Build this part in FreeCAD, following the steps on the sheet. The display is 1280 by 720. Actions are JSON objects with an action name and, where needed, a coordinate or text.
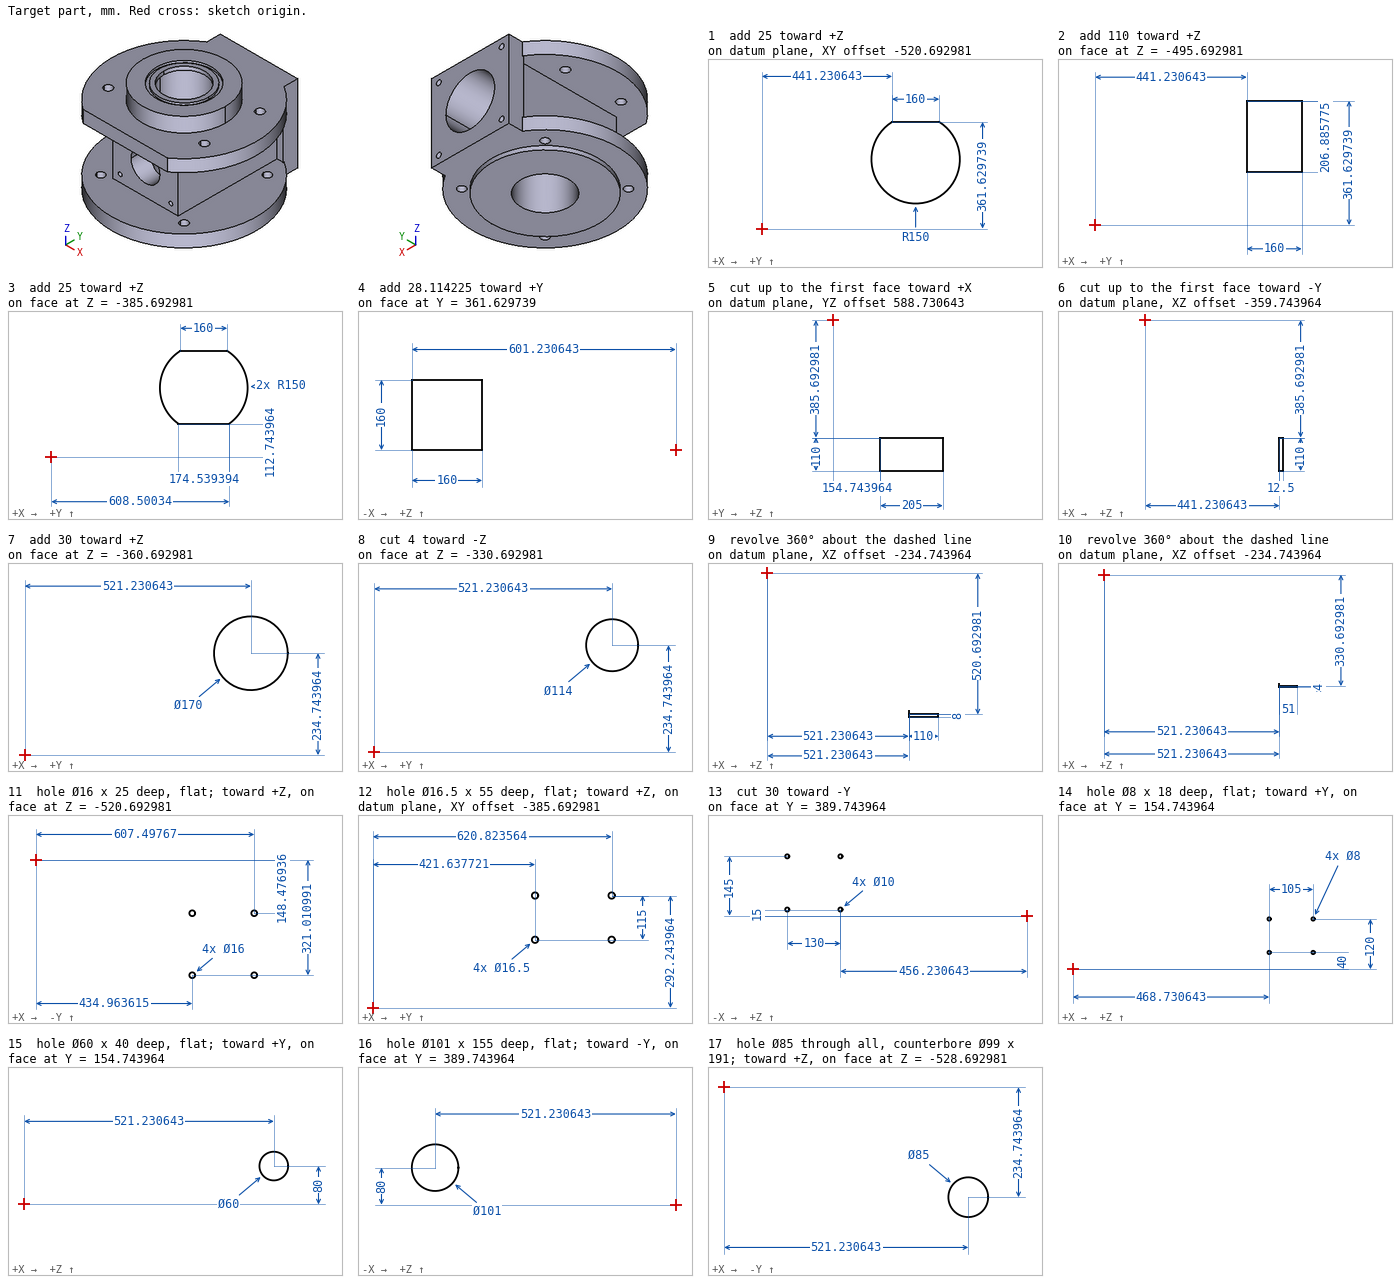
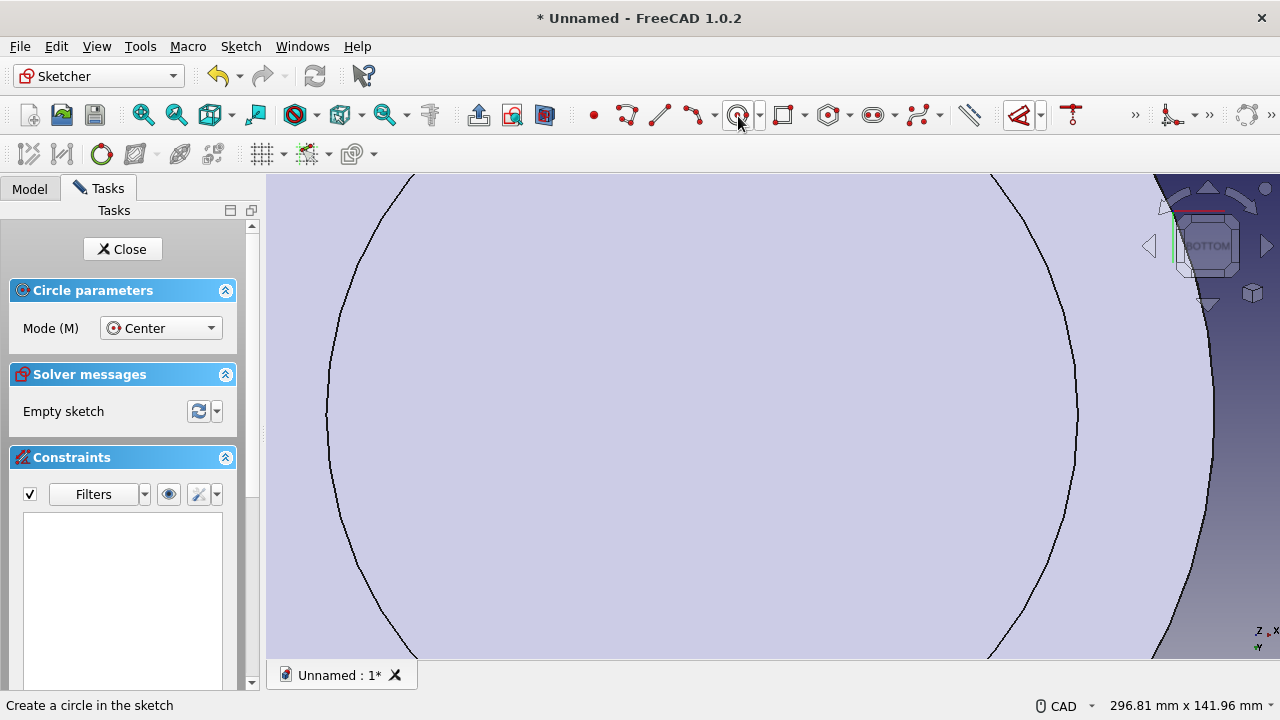
{"action": "left_click", "coordinate": [702, 415]}
{"action": "left_click", "coordinate": [805, 312]}
{"action": "key", "text": "Escape"}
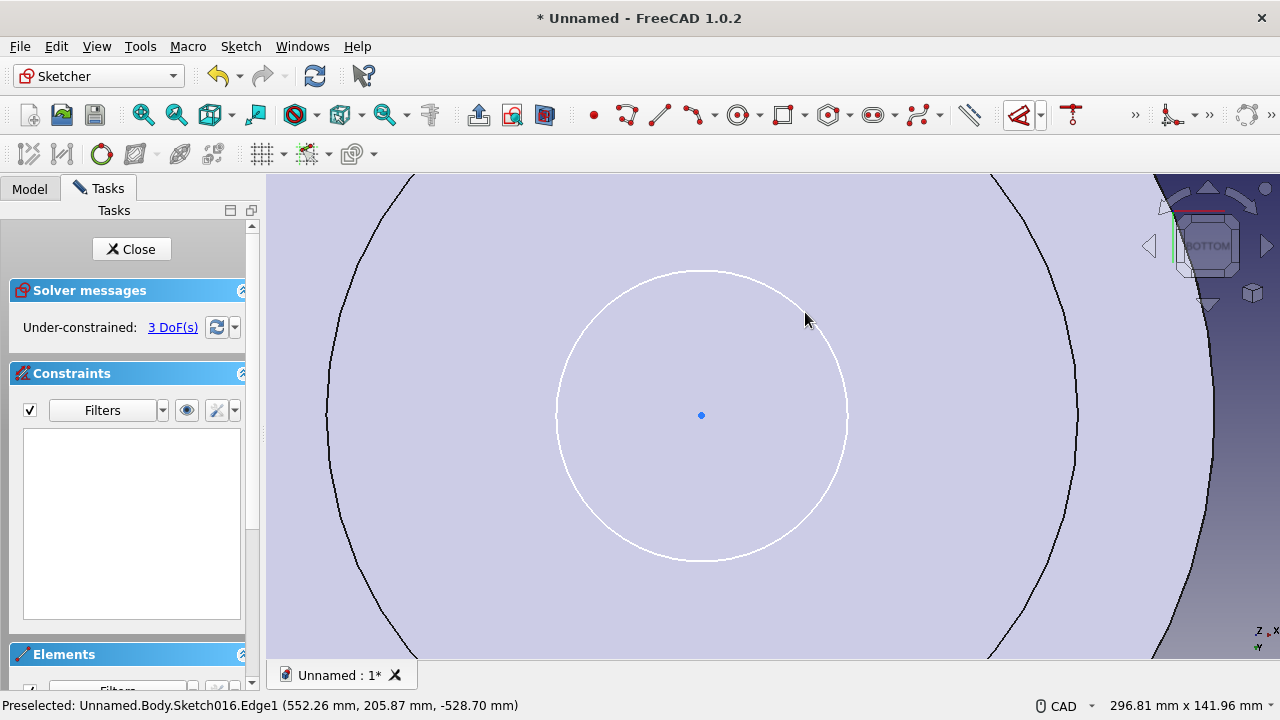
{"action": "left_click", "coordinate": [805, 313]}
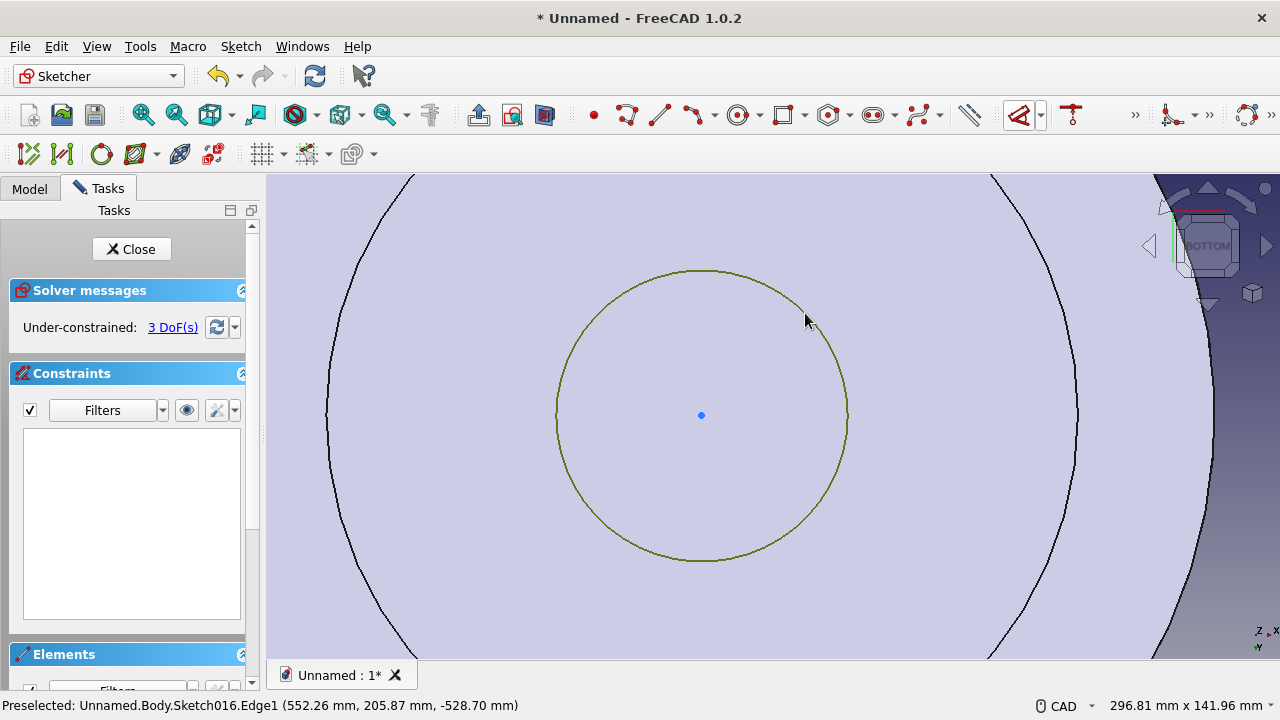
{"action": "key", "text": "k o"}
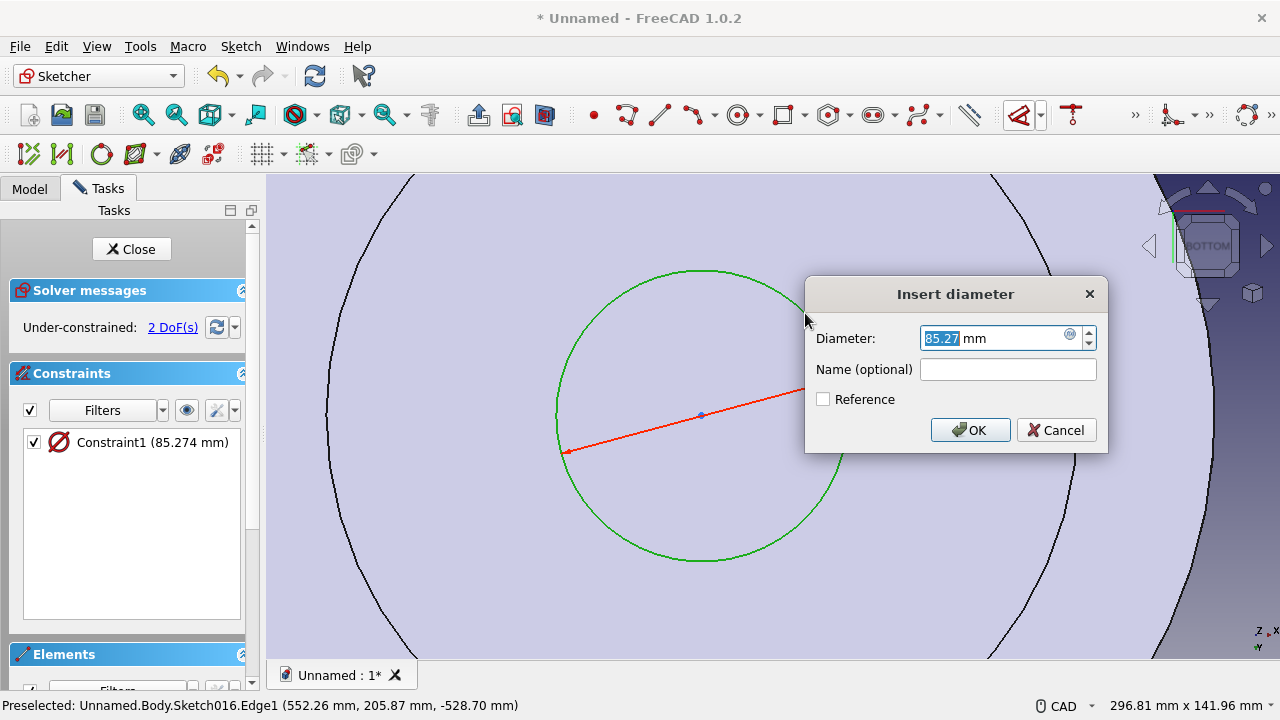
{"action": "type", "text": "85"}
{"action": "key", "text": "Return"}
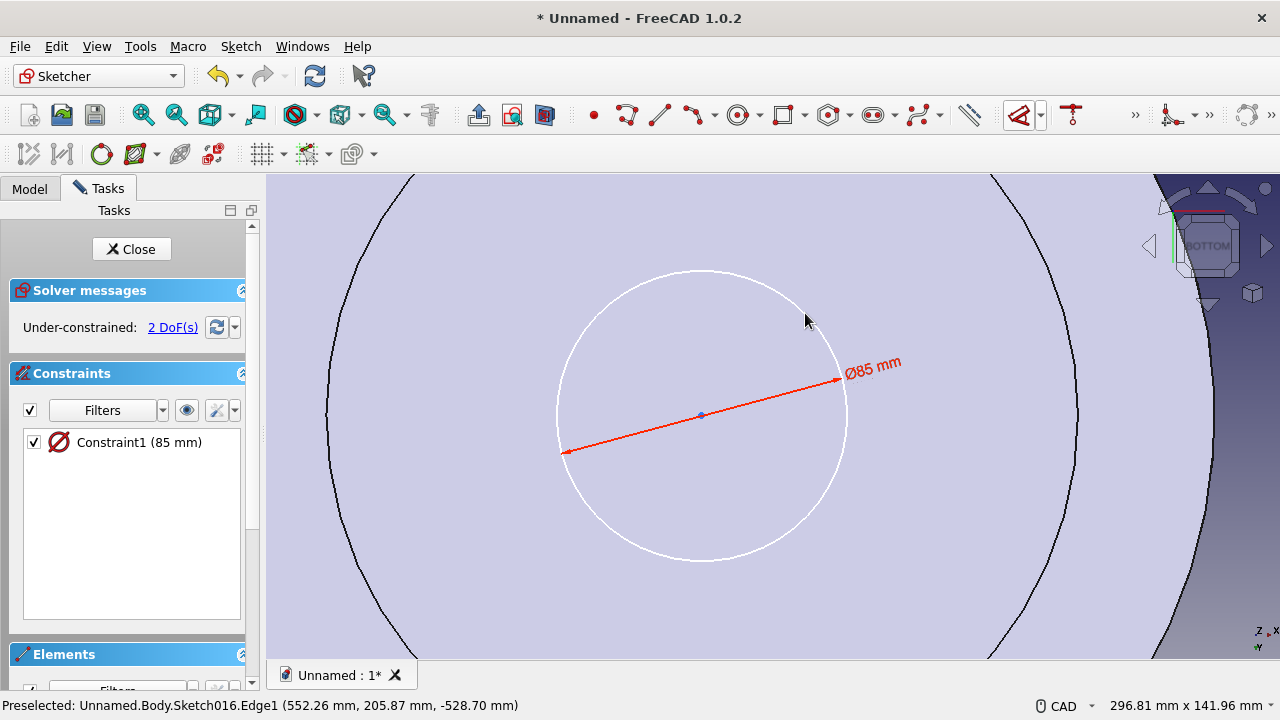
{"action": "left_click", "coordinate": [702, 416]}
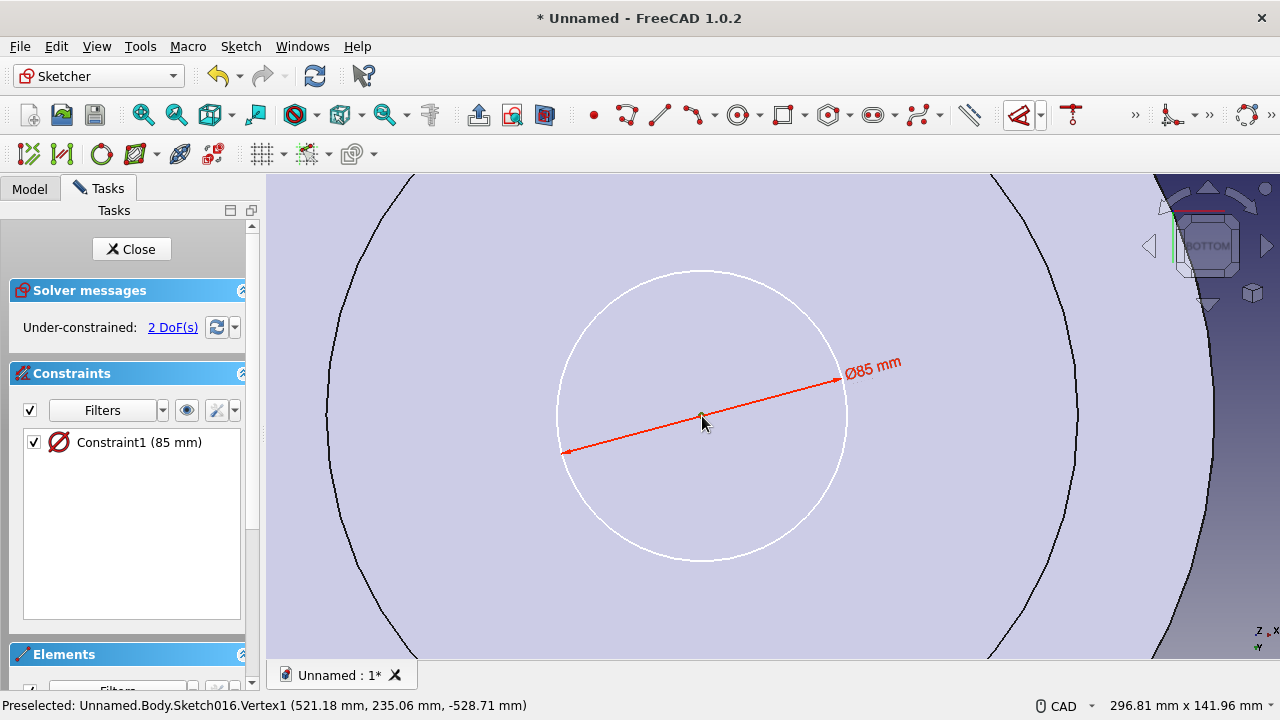
{"action": "key", "text": "l"}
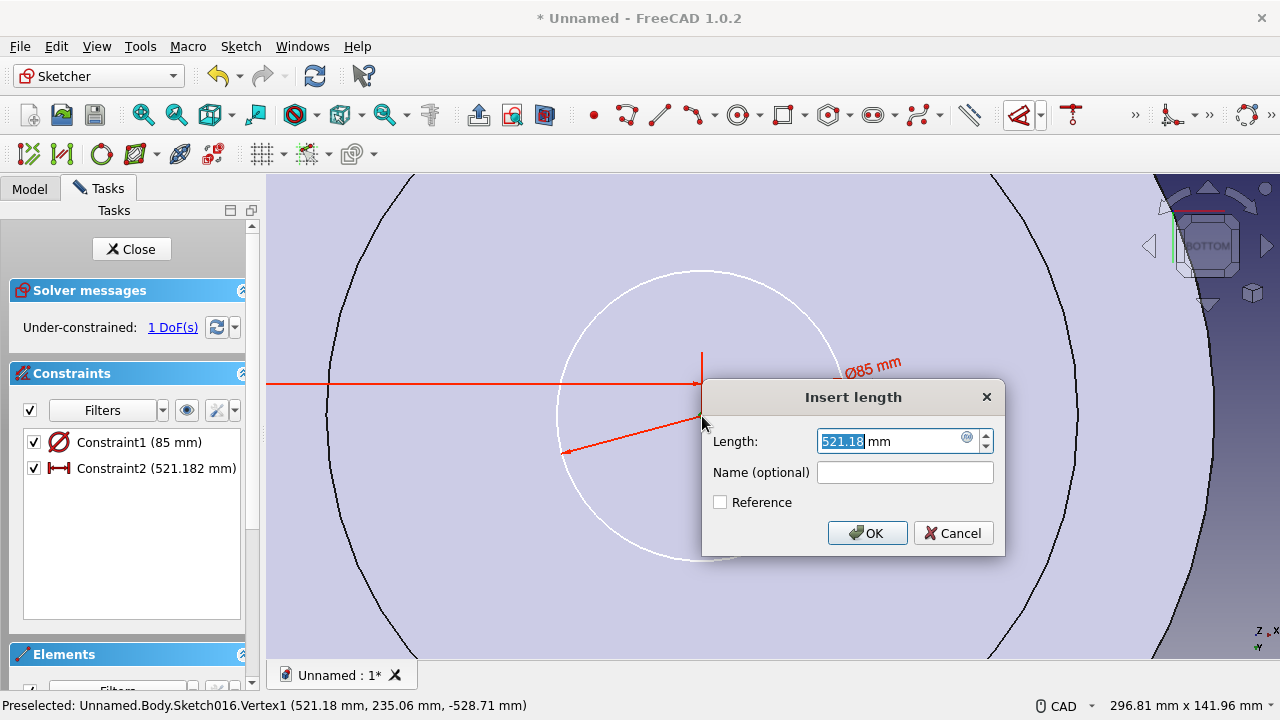
{"action": "type", "text": "521.230643"}
{"action": "key", "text": "Return"}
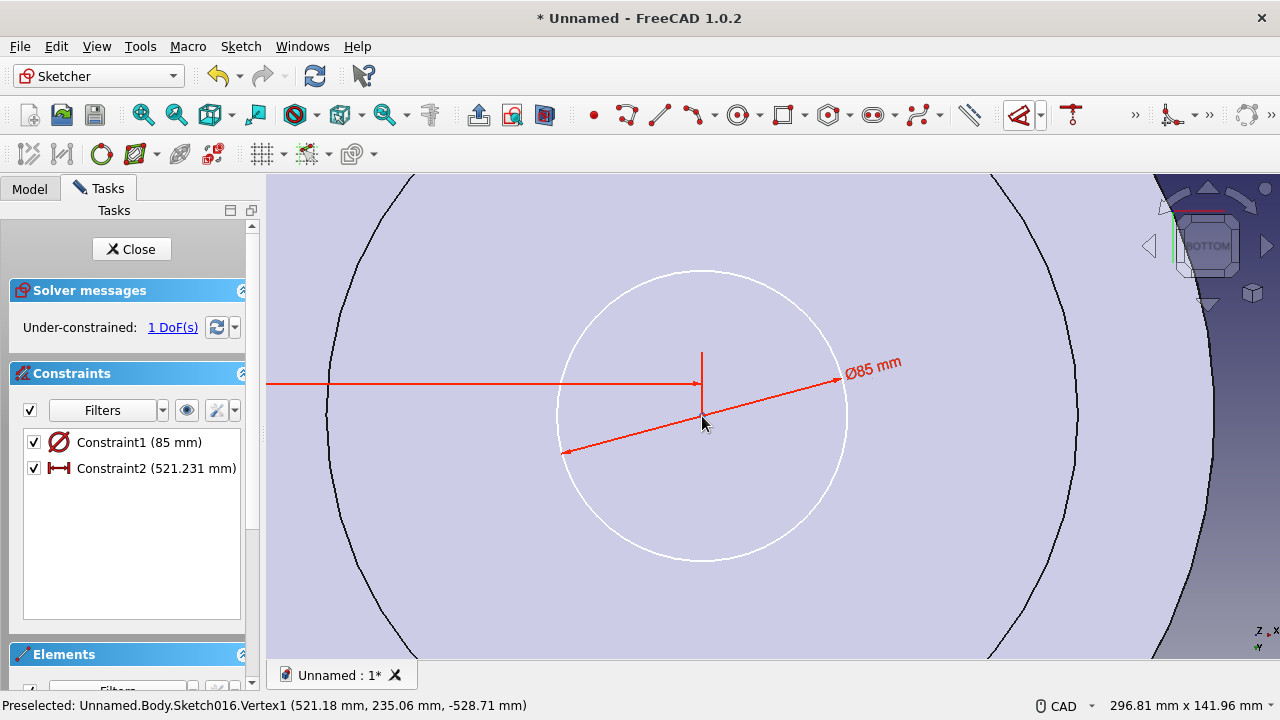
{"action": "left_click", "coordinate": [702, 416]}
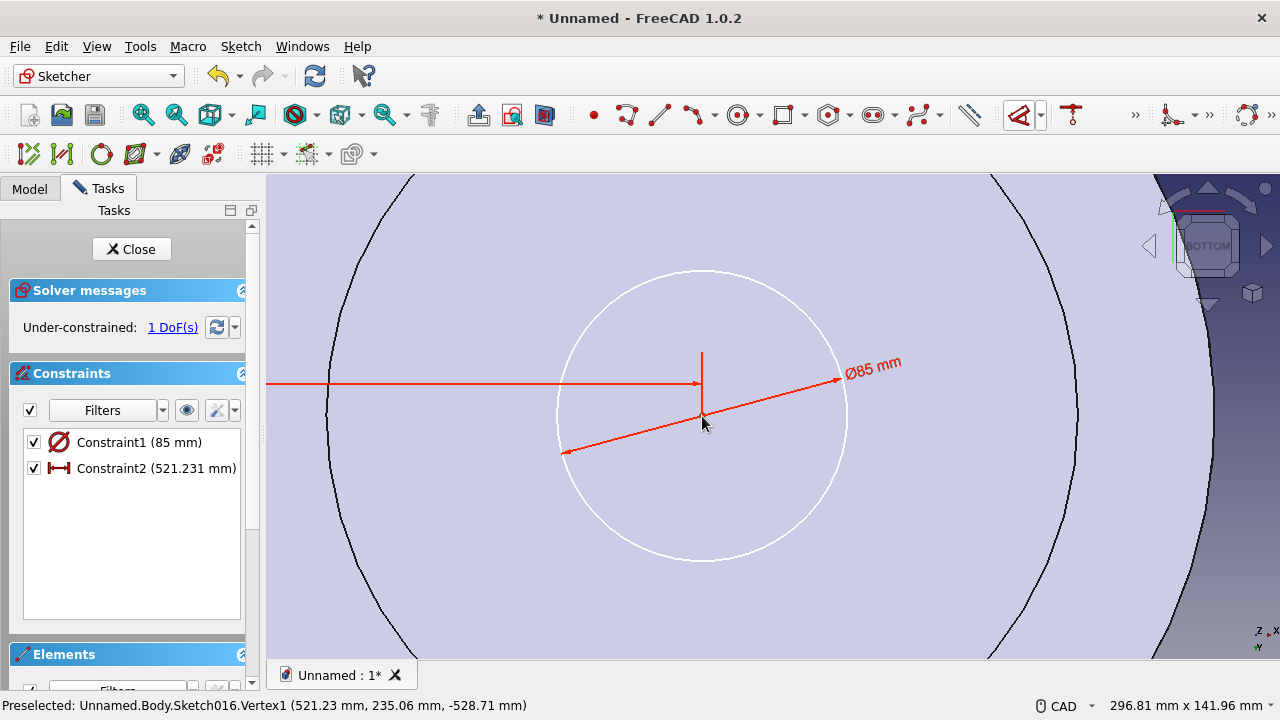
{"action": "left_click", "coordinate": [1040, 116]}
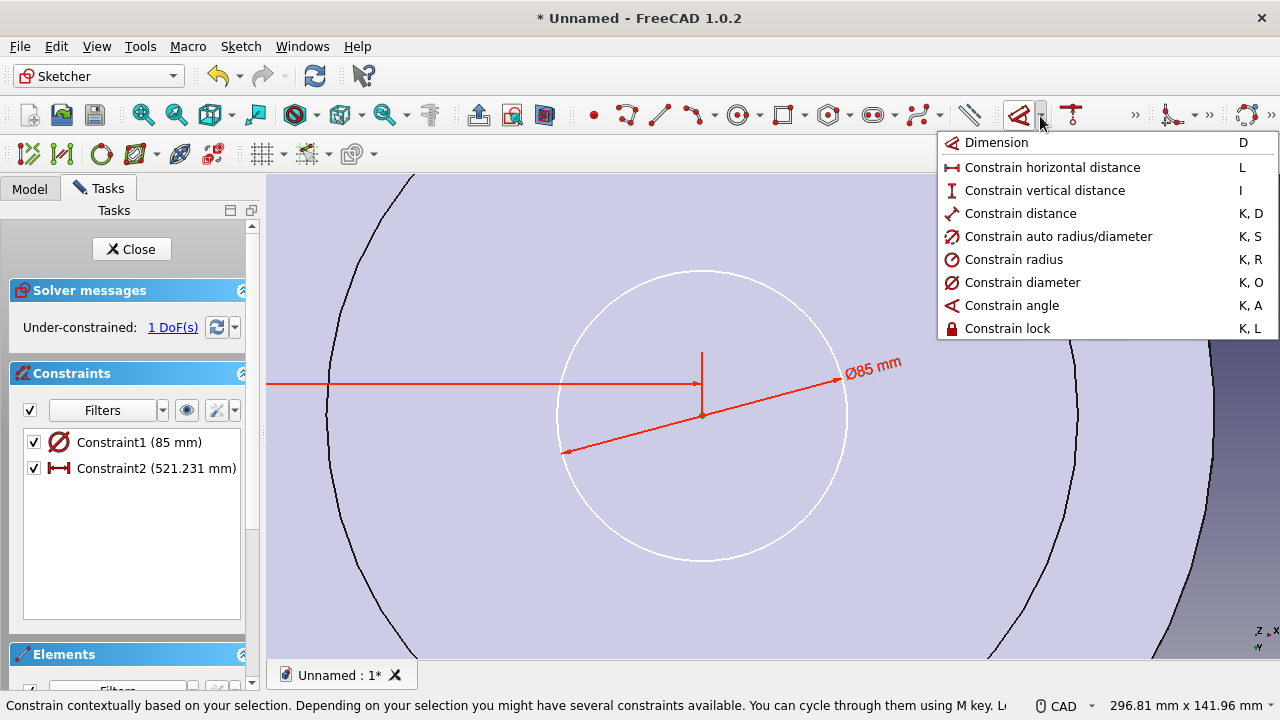
{"action": "left_click", "coordinate": [1108, 190]}